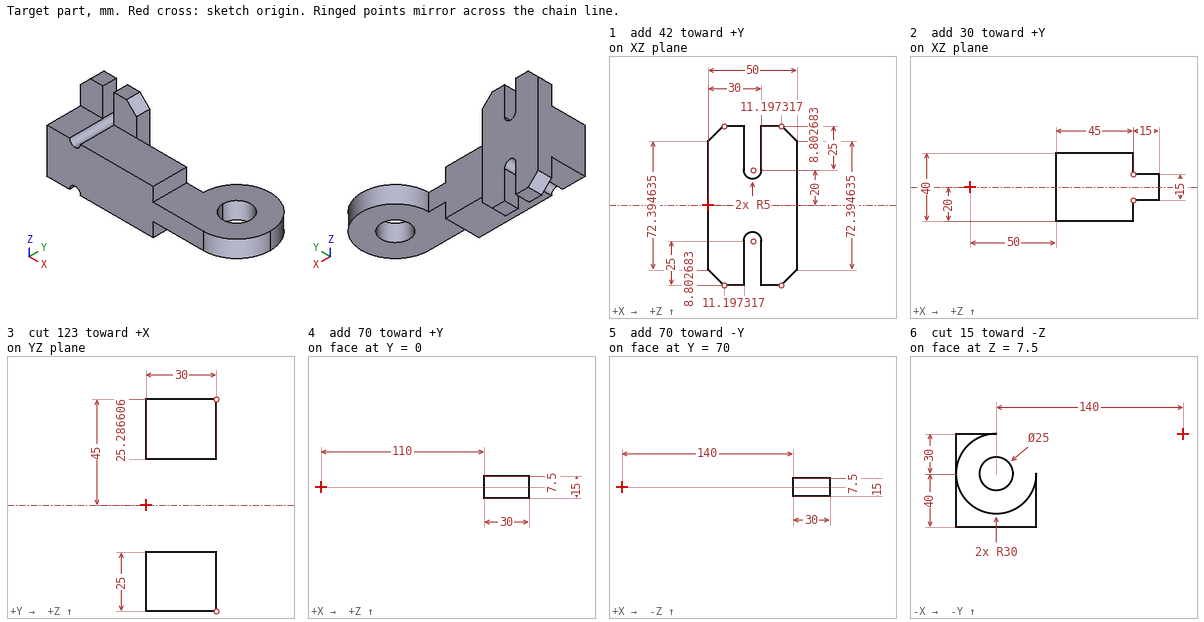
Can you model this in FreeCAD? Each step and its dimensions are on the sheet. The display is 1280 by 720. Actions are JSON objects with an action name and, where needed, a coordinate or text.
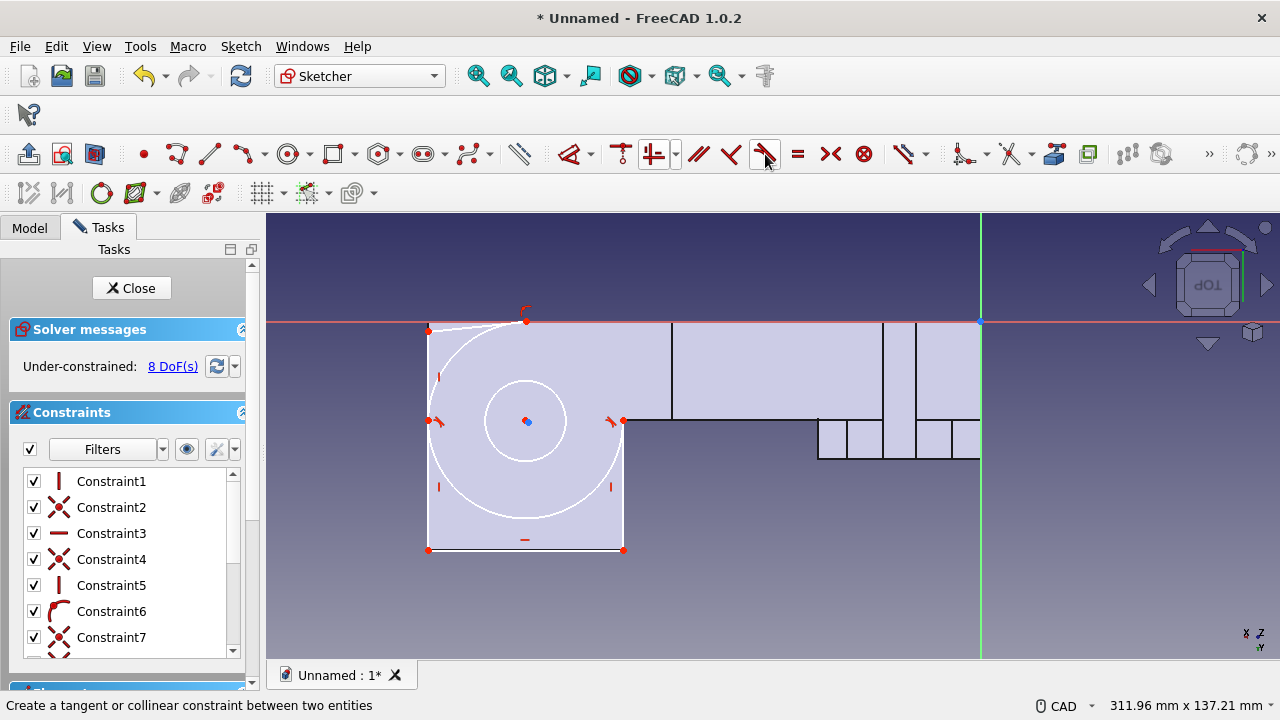
{"action": "left_click", "coordinate": [468, 500]}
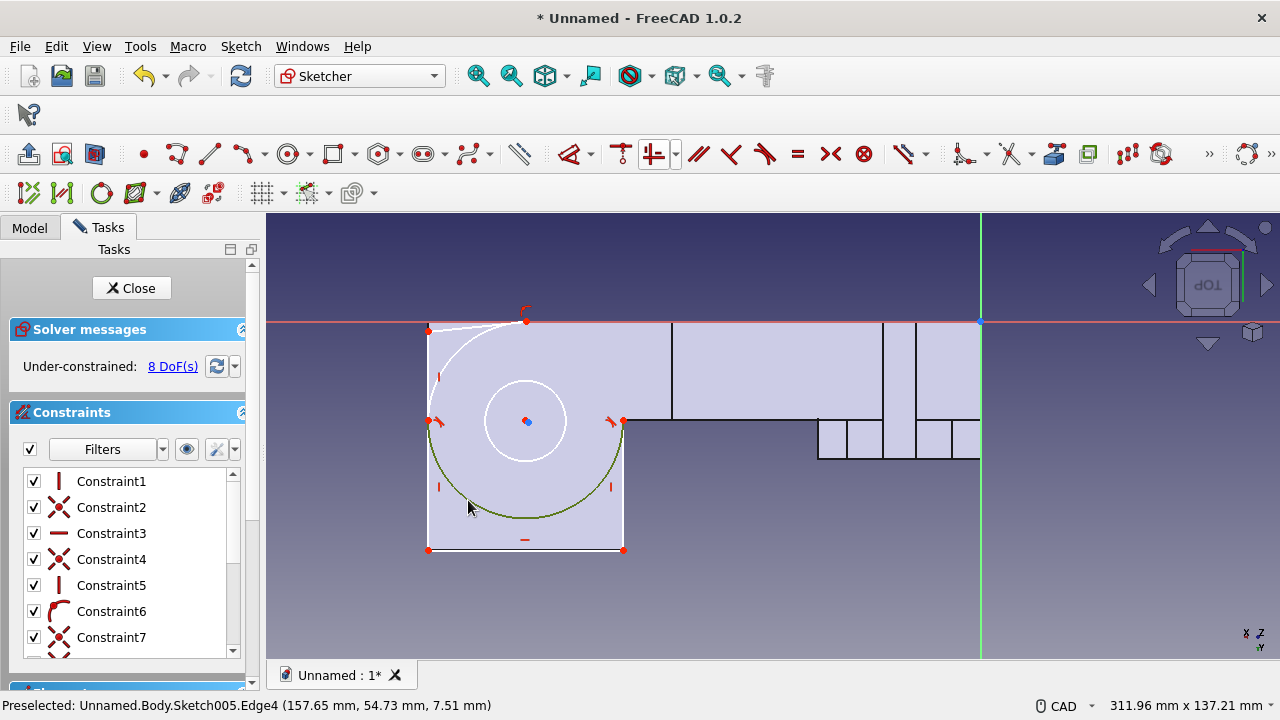
{"action": "scroll", "coordinate": [439, 377], "scroll_direction": "up", "scroll_amount": 2}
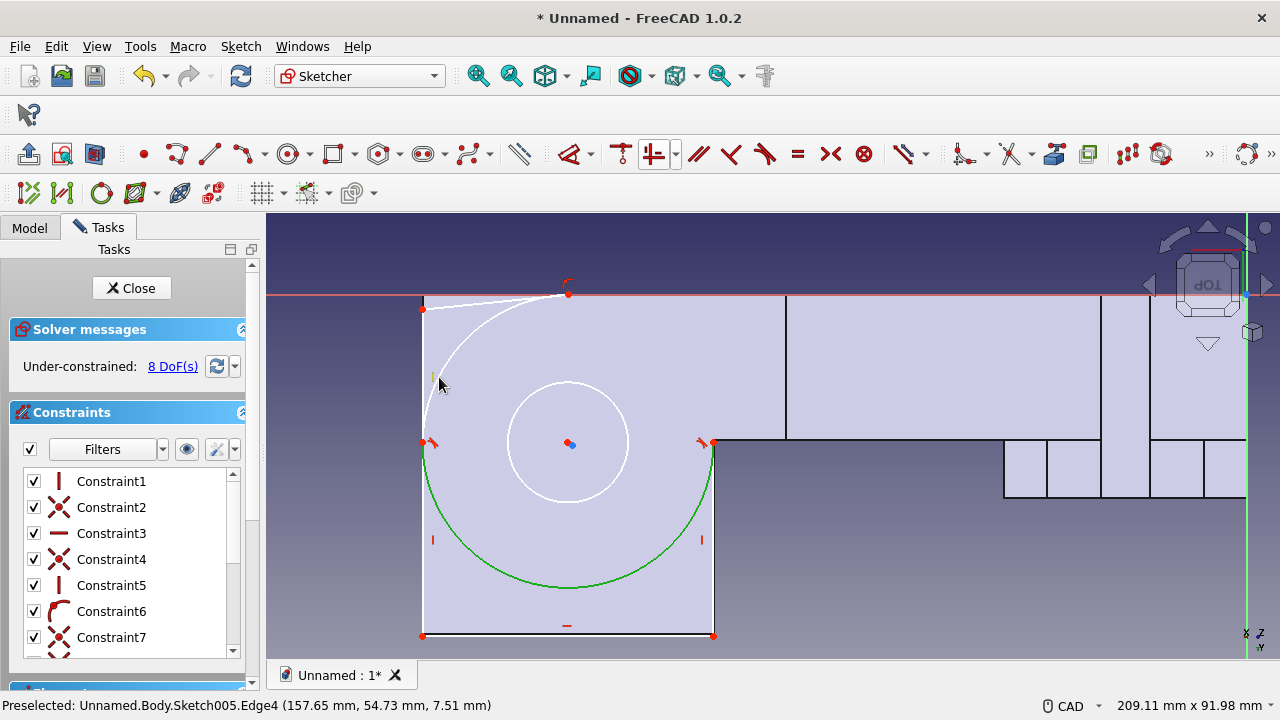
{"action": "left_click", "coordinate": [466, 339]}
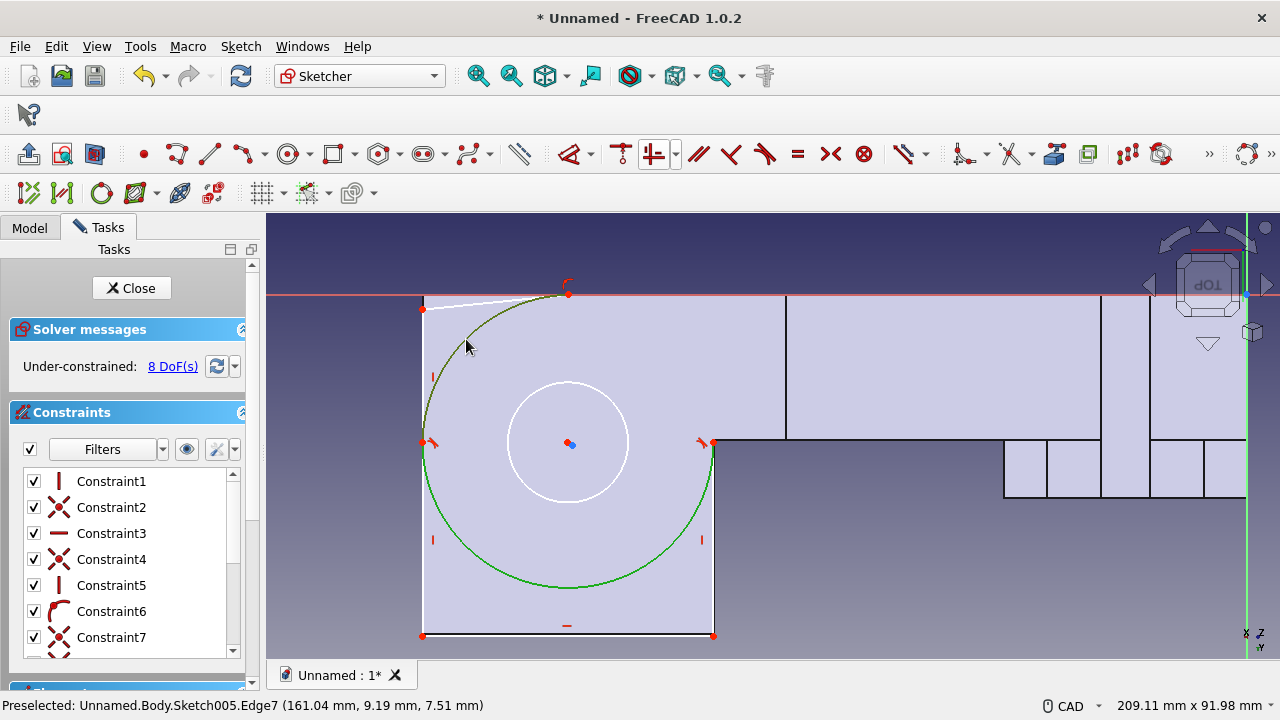
{"action": "key", "text": "t"}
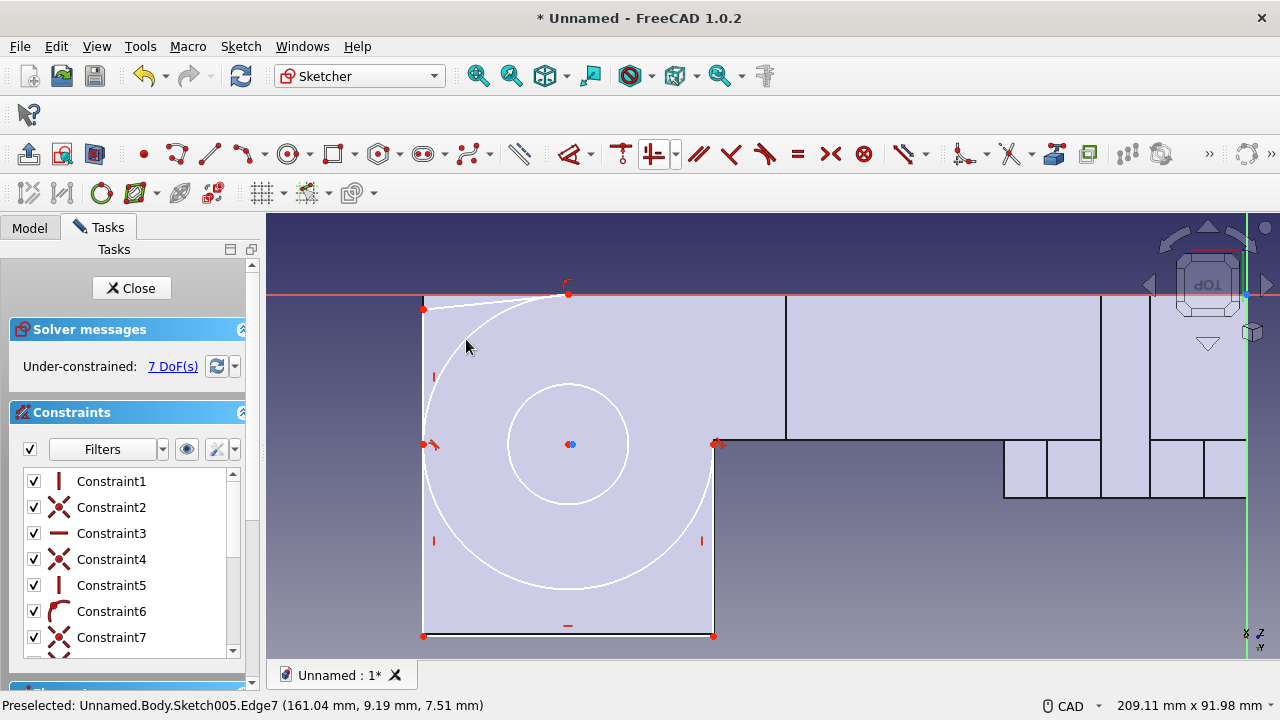
{"action": "scroll", "coordinate": [467, 305], "scroll_direction": "up", "scroll_amount": 2}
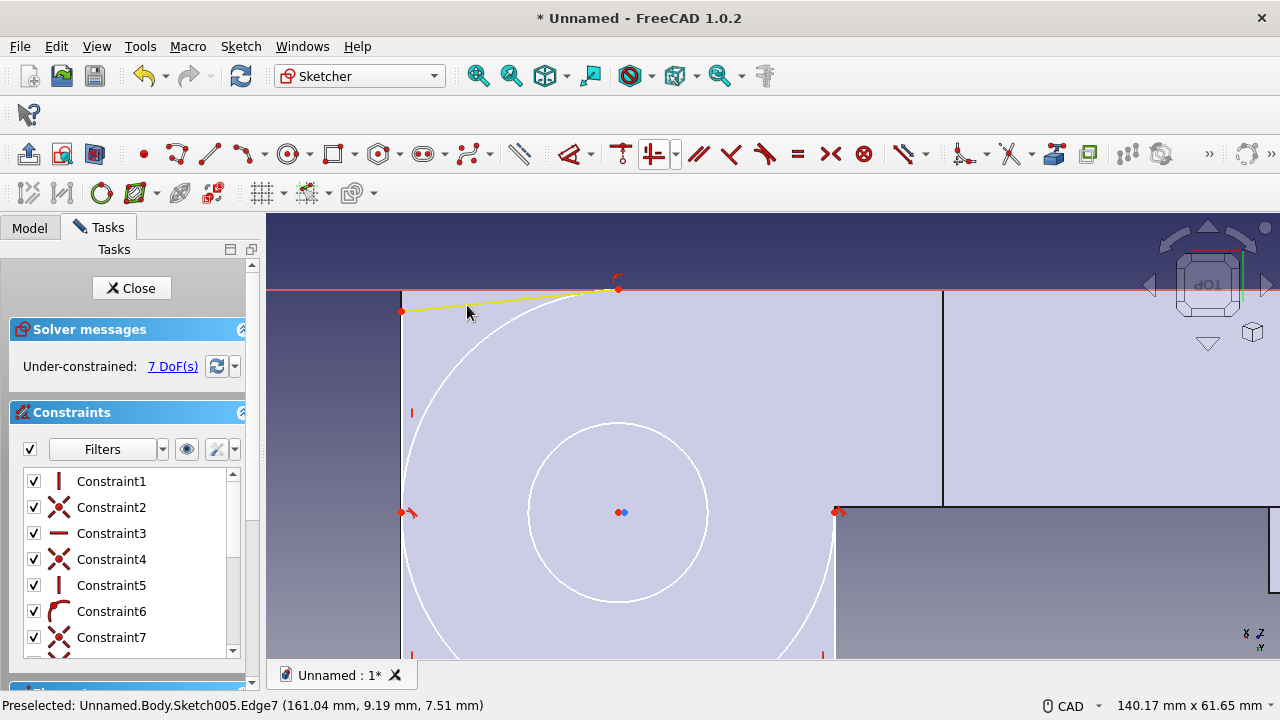
{"action": "left_click", "coordinate": [467, 305]}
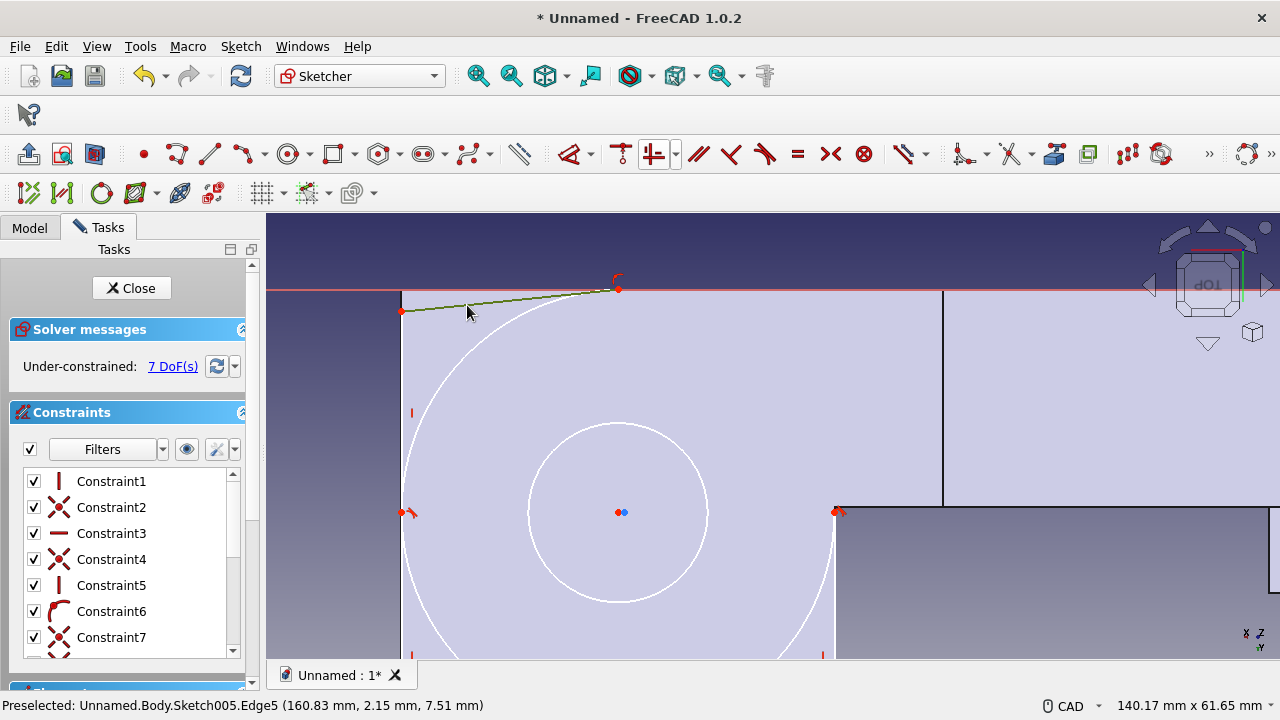
{"action": "left_click", "coordinate": [520, 316]}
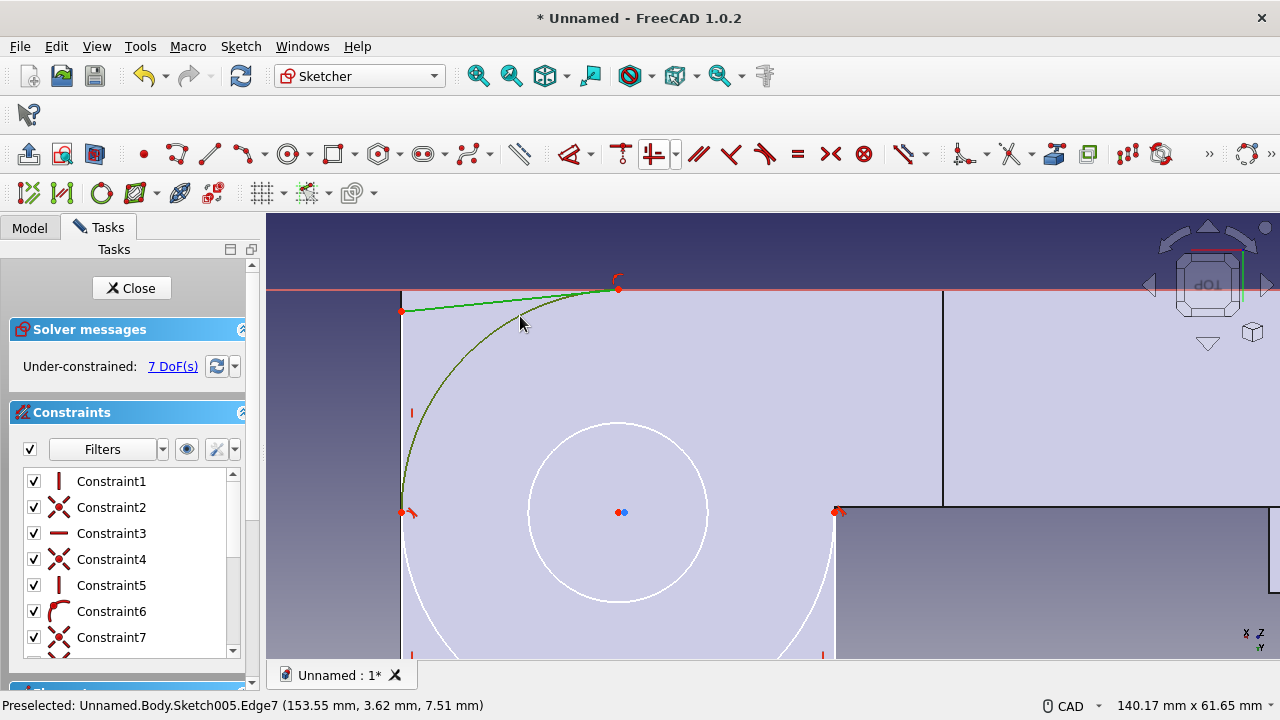
{"action": "key", "text": "t"}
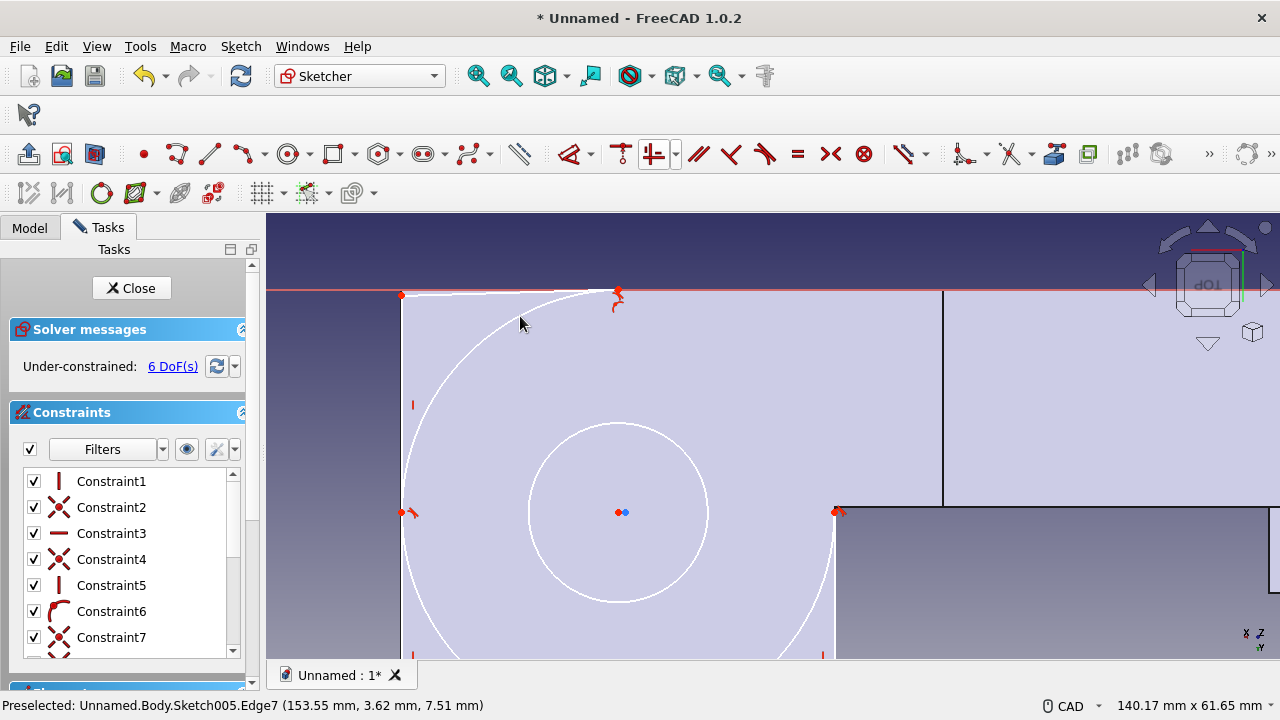
{"action": "scroll", "coordinate": [554, 292], "scroll_direction": "up", "scroll_amount": 2}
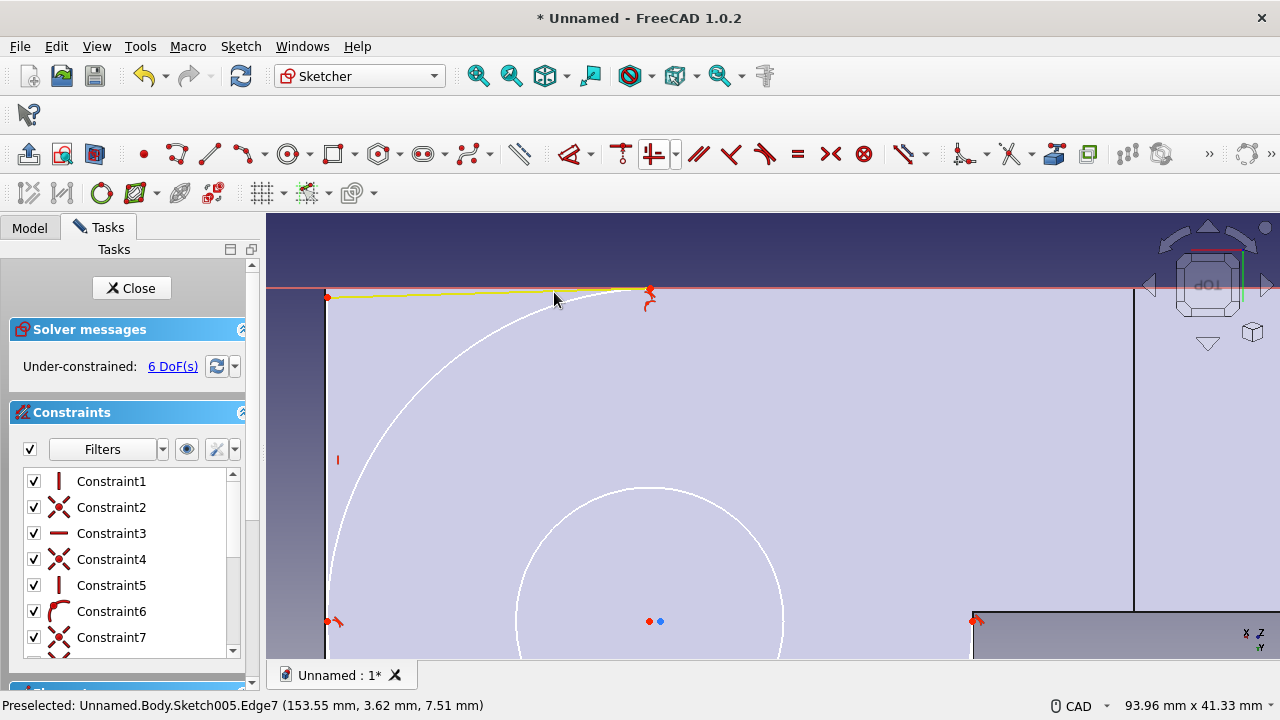
{"action": "left_click", "coordinate": [553, 291]}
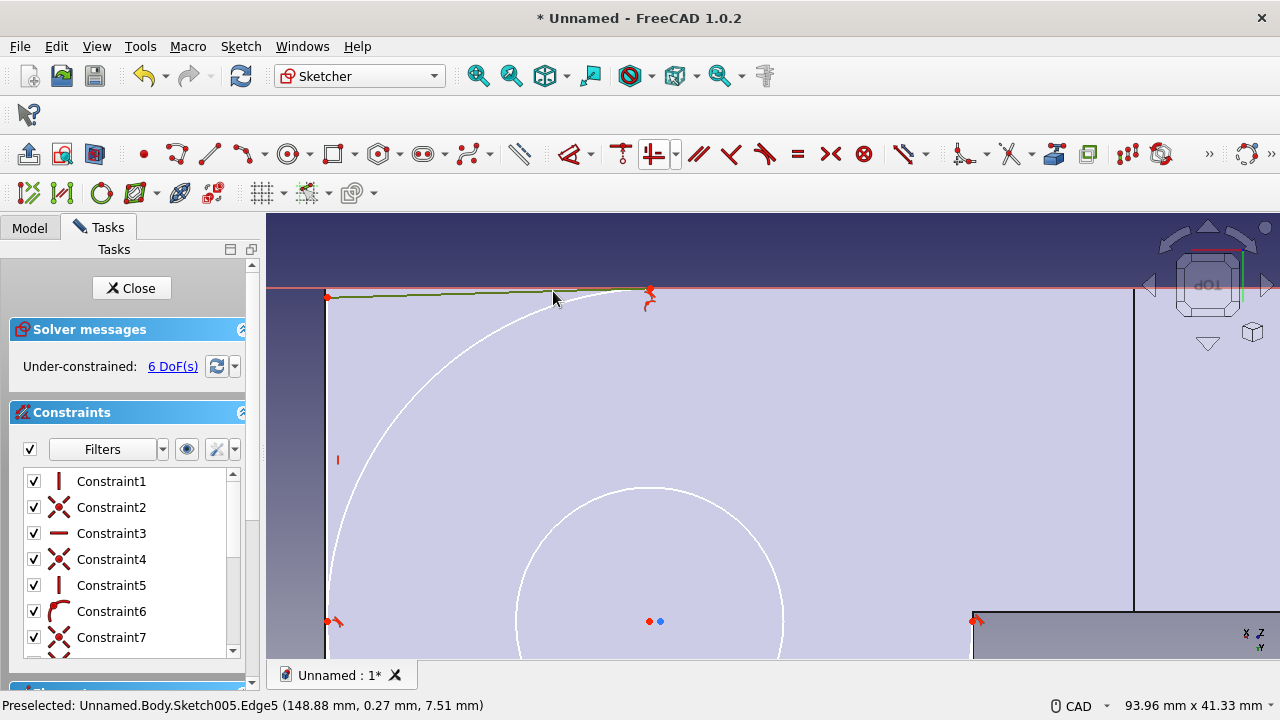
{"action": "key", "text": "h"}